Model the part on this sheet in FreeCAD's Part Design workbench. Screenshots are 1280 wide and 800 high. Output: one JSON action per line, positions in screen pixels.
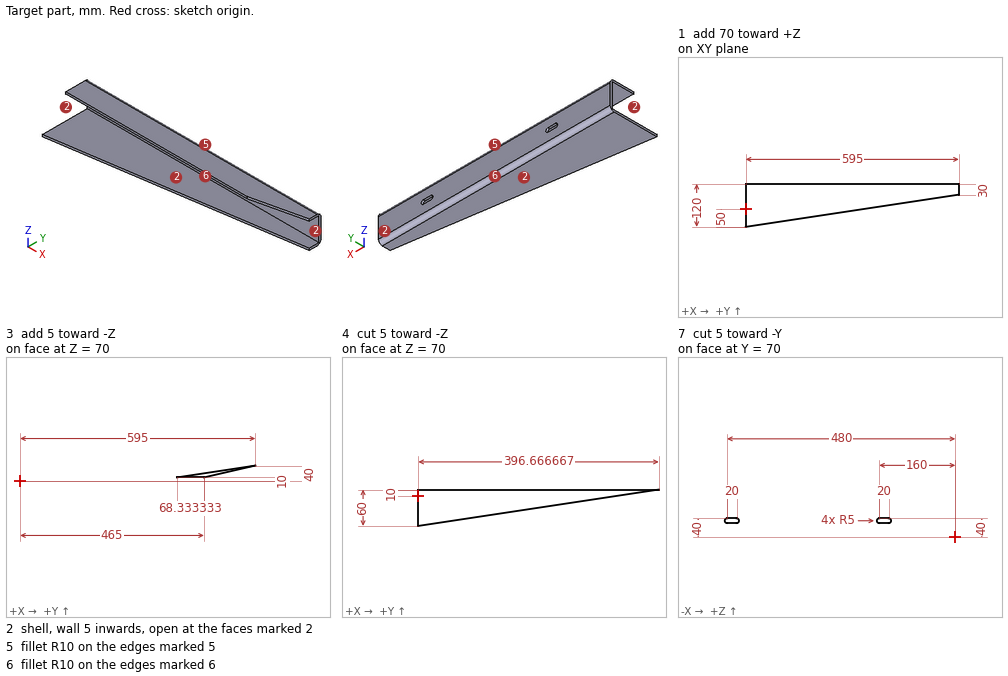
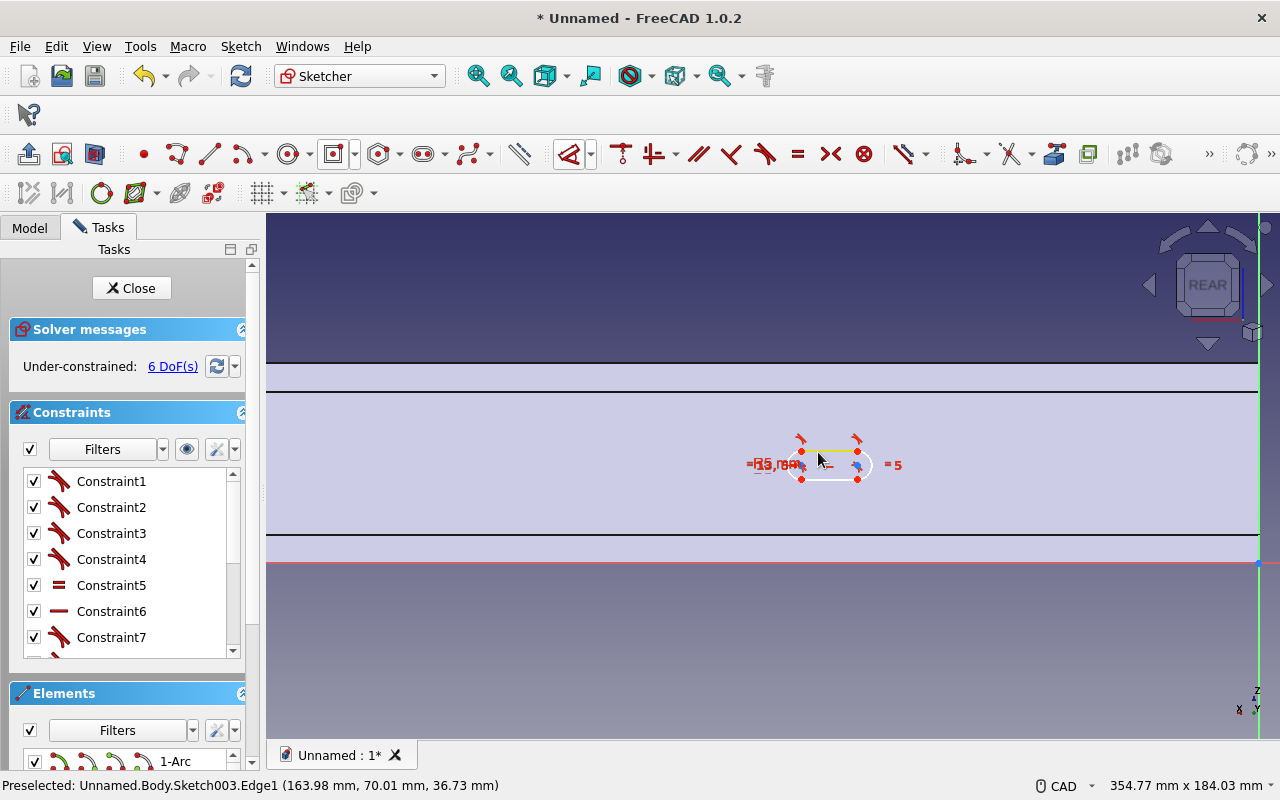
{"action": "left_click", "coordinate": [818, 451]}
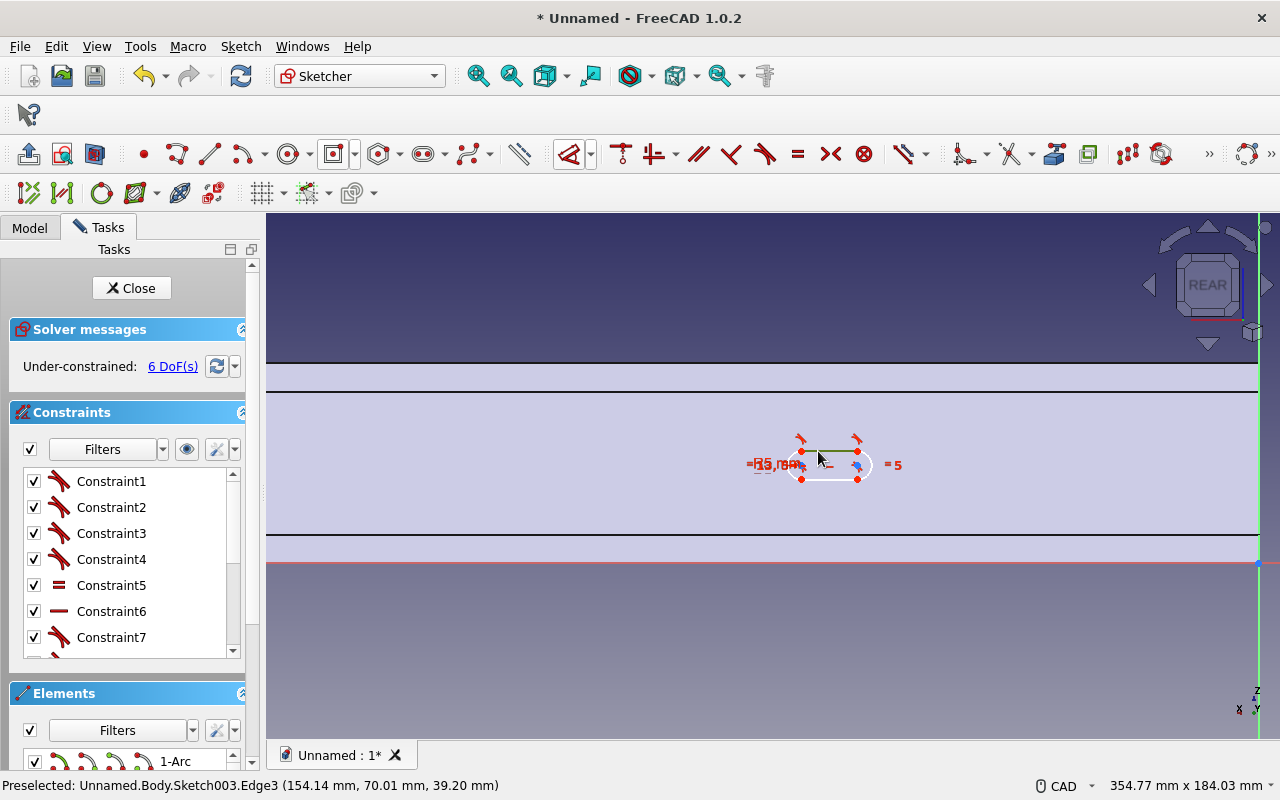
{"action": "key", "text": "l"}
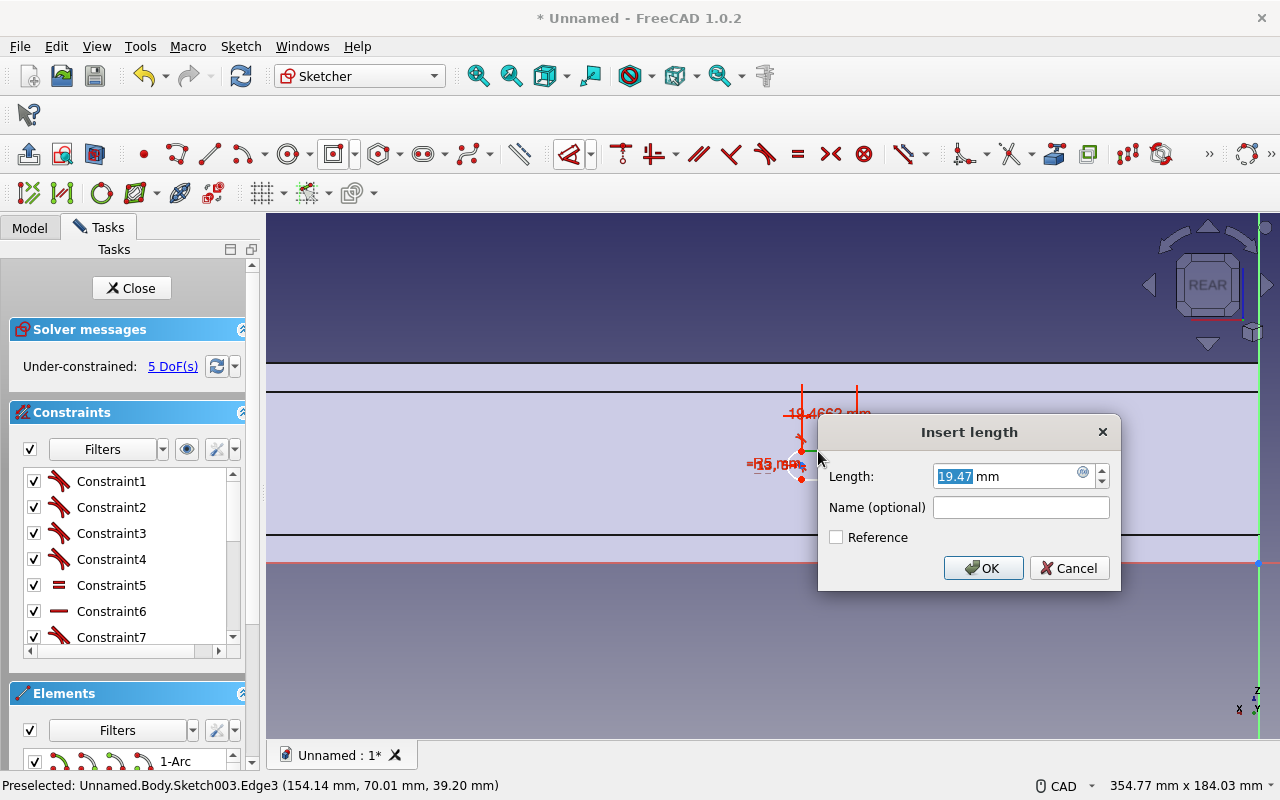
{"action": "type", "text": "20"}
{"action": "key", "text": "Return"}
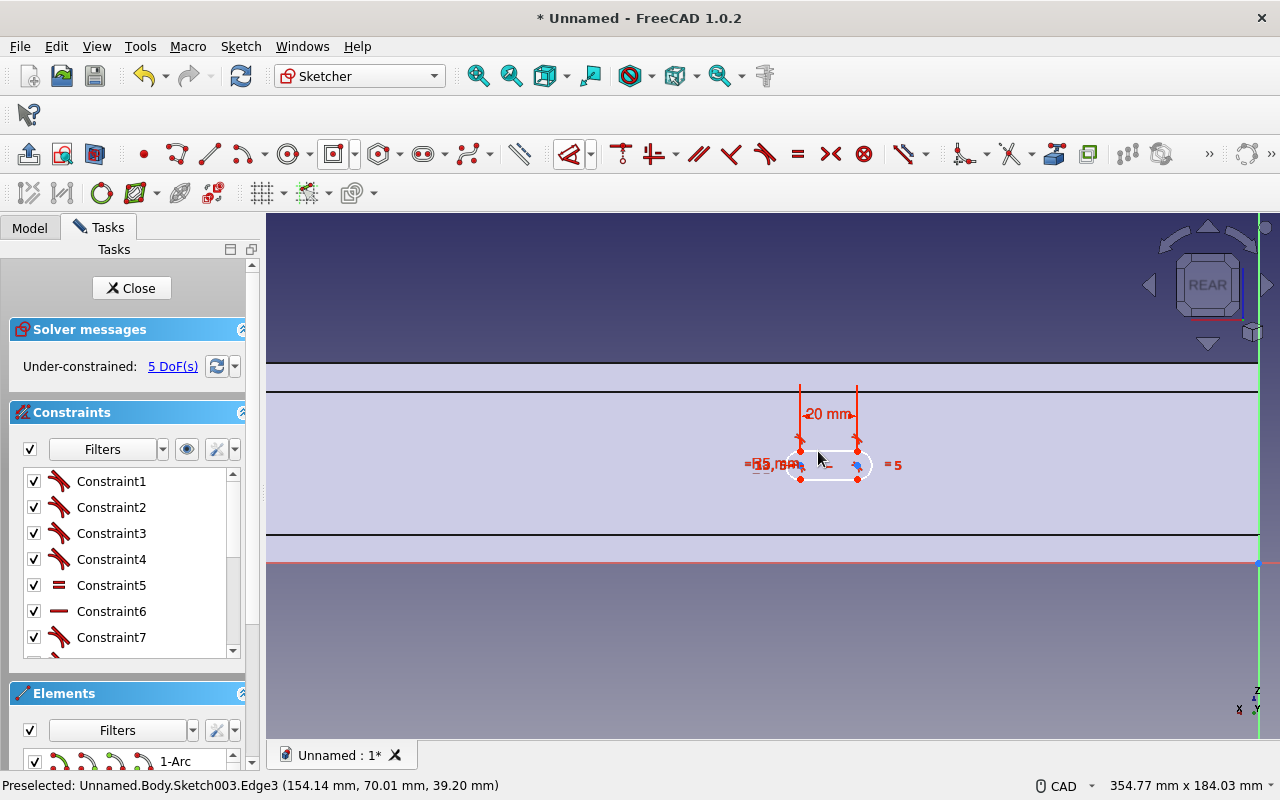
{"action": "scroll", "coordinate": [818, 451], "scroll_direction": "down", "scroll_amount": 4}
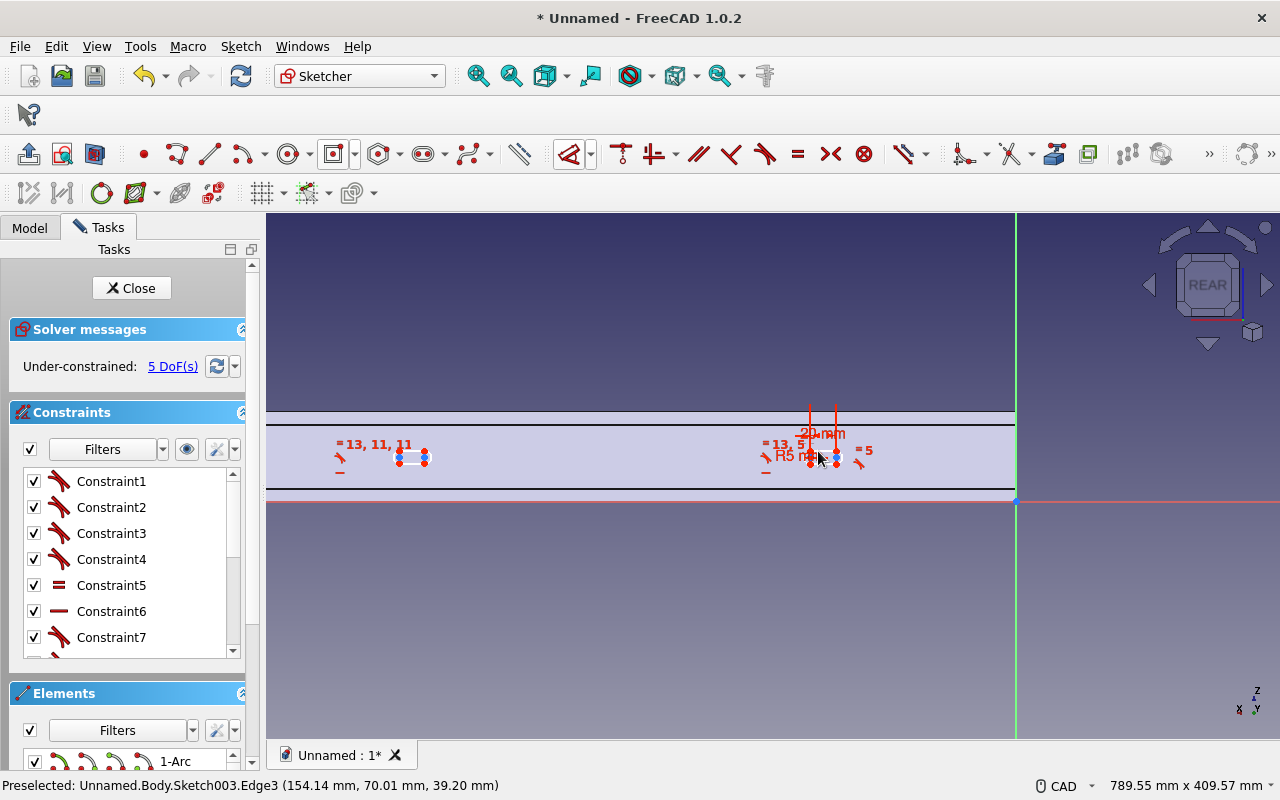
{"action": "scroll", "coordinate": [408, 451], "scroll_direction": "up", "scroll_amount": 4}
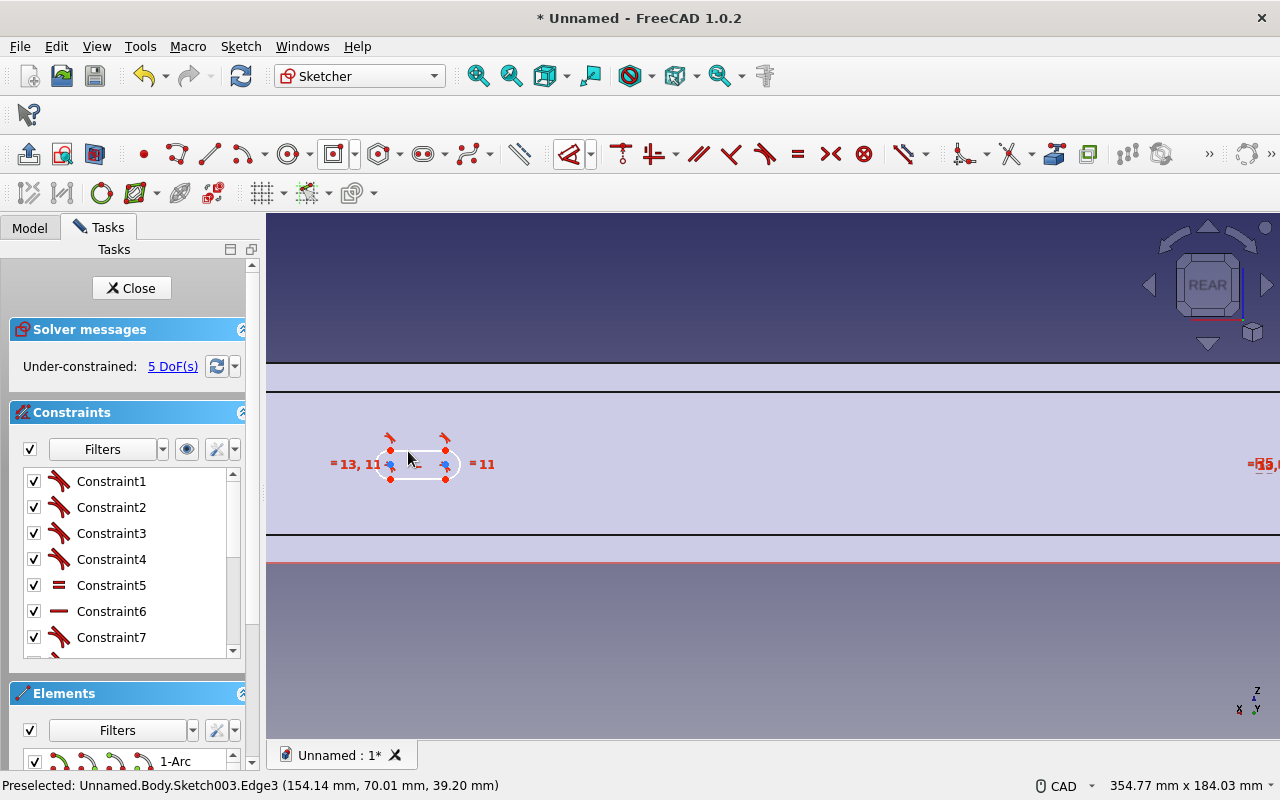
{"action": "left_click", "coordinate": [407, 451]}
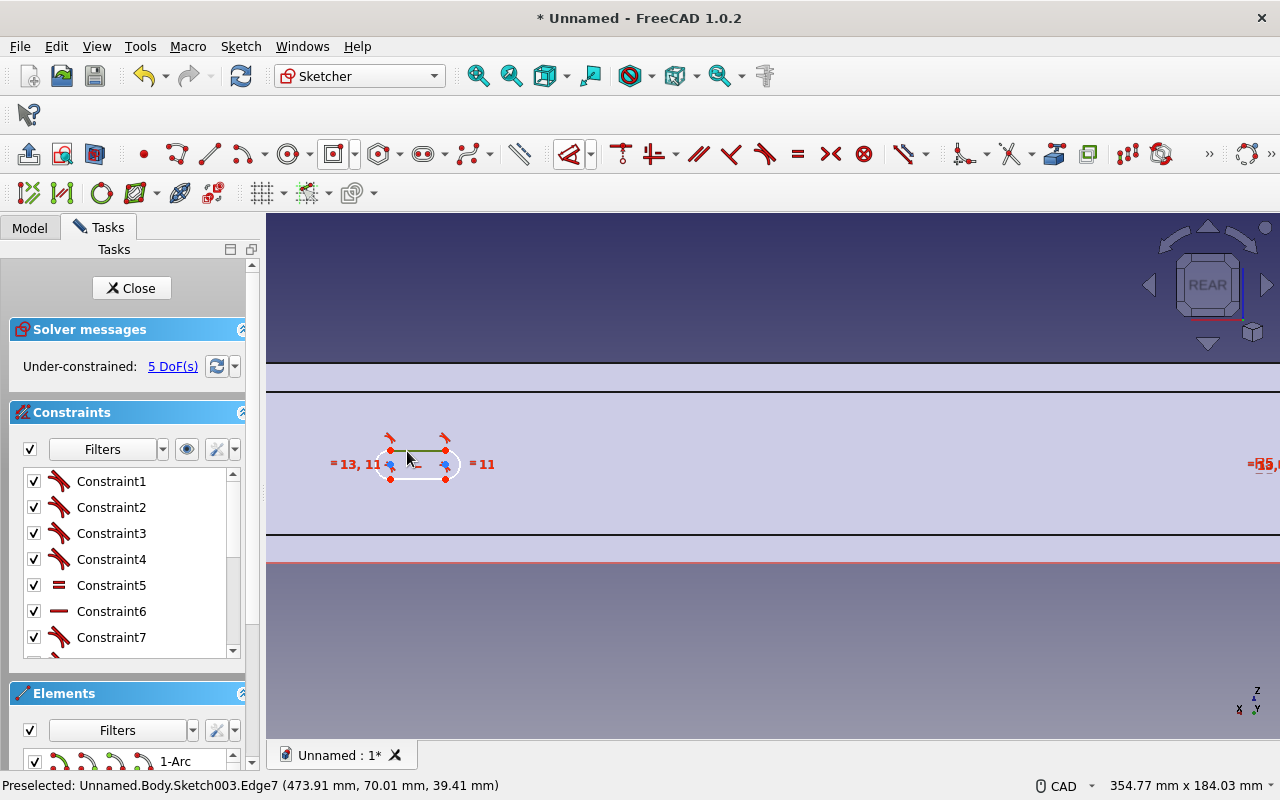
{"action": "key", "text": "l"}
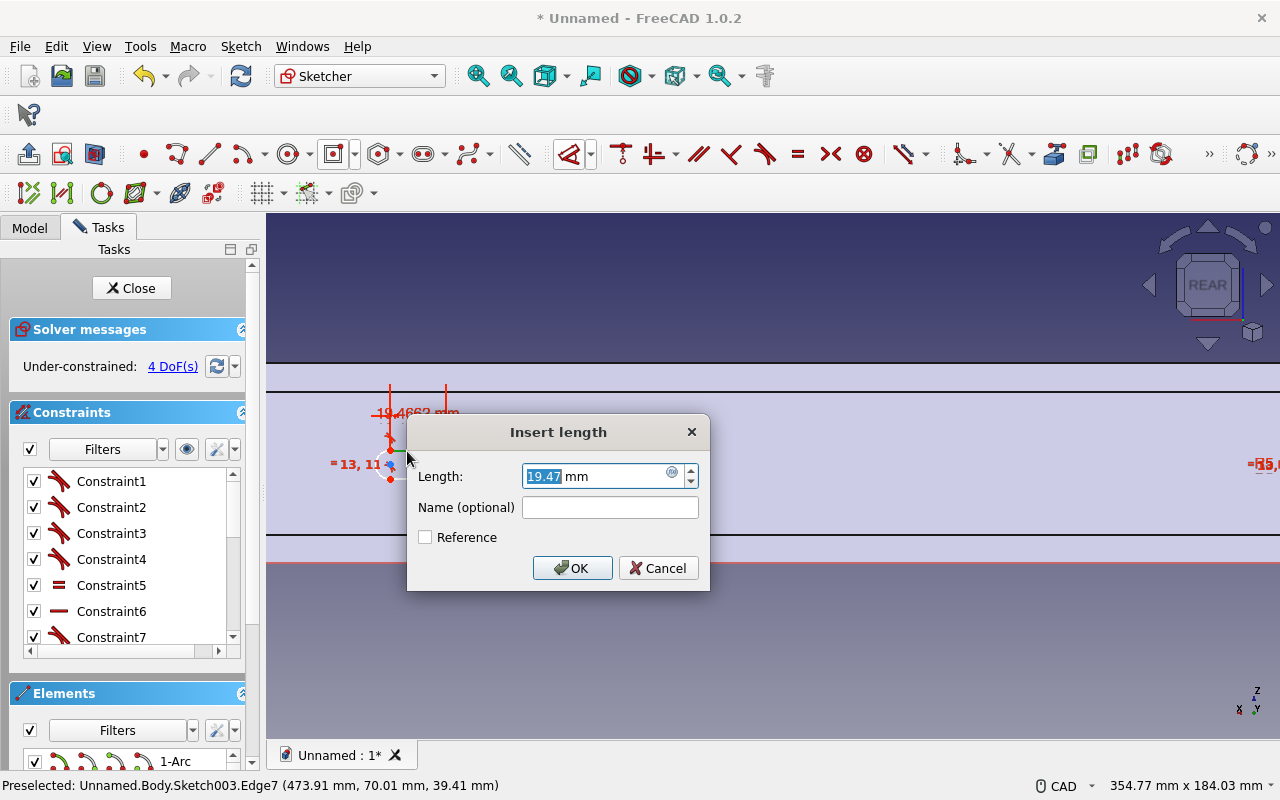
{"action": "type", "text": "20"}
{"action": "key", "text": "Return"}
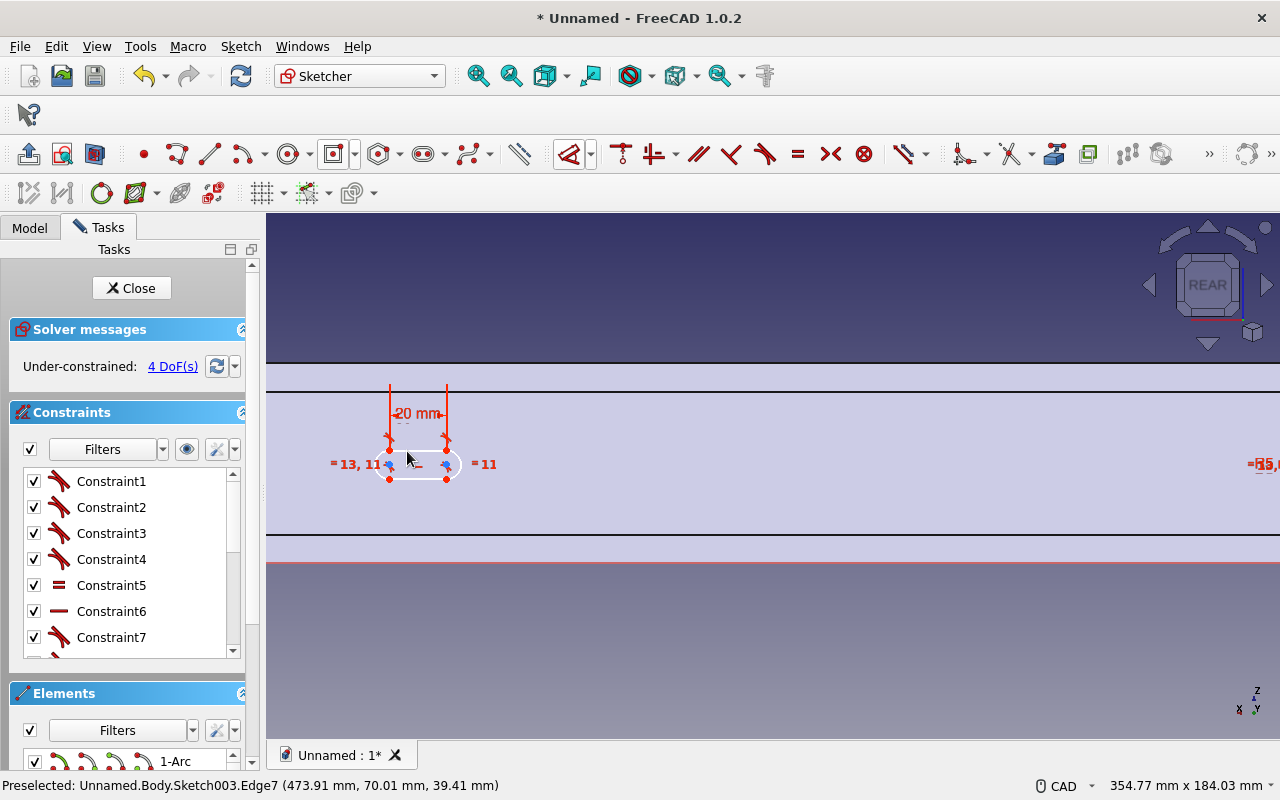
{"action": "scroll", "coordinate": [408, 451], "scroll_direction": "down", "scroll_amount": 4}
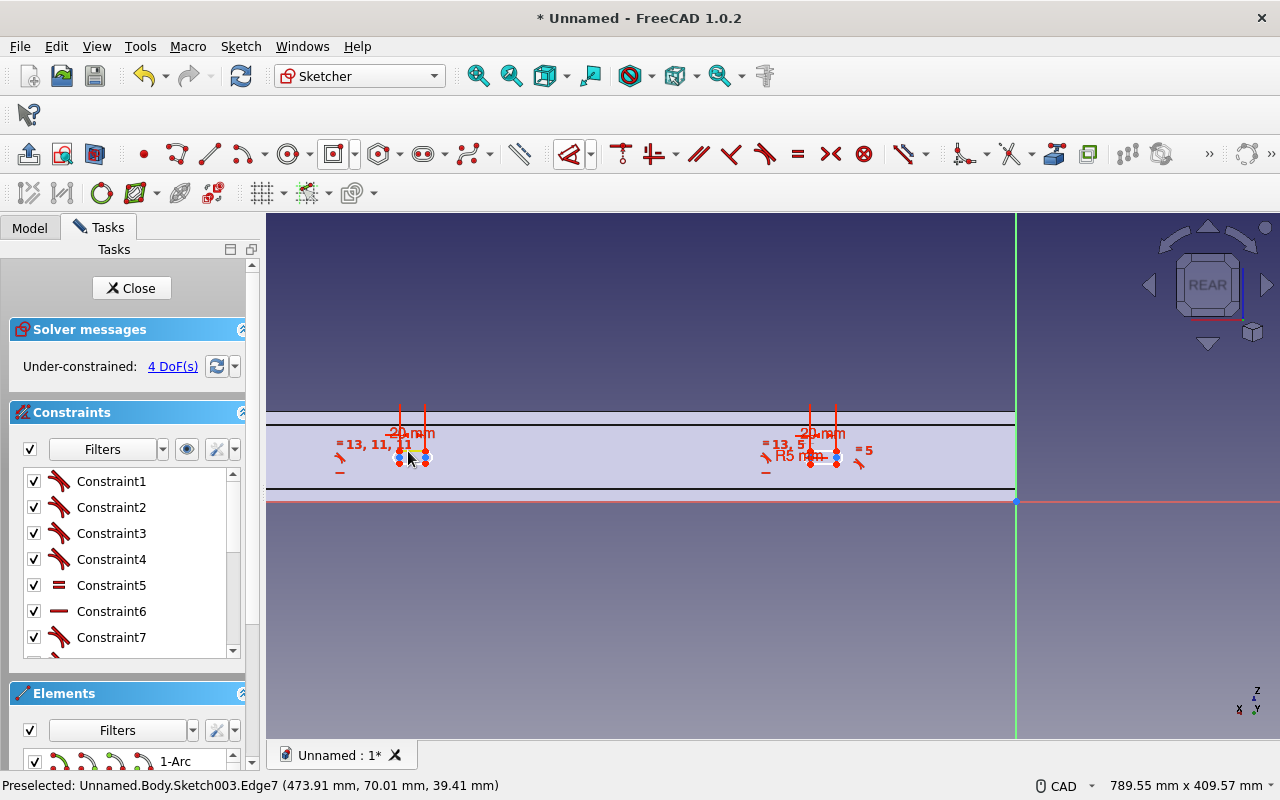
{"action": "scroll", "coordinate": [810, 451], "scroll_direction": "up", "scroll_amount": 4}